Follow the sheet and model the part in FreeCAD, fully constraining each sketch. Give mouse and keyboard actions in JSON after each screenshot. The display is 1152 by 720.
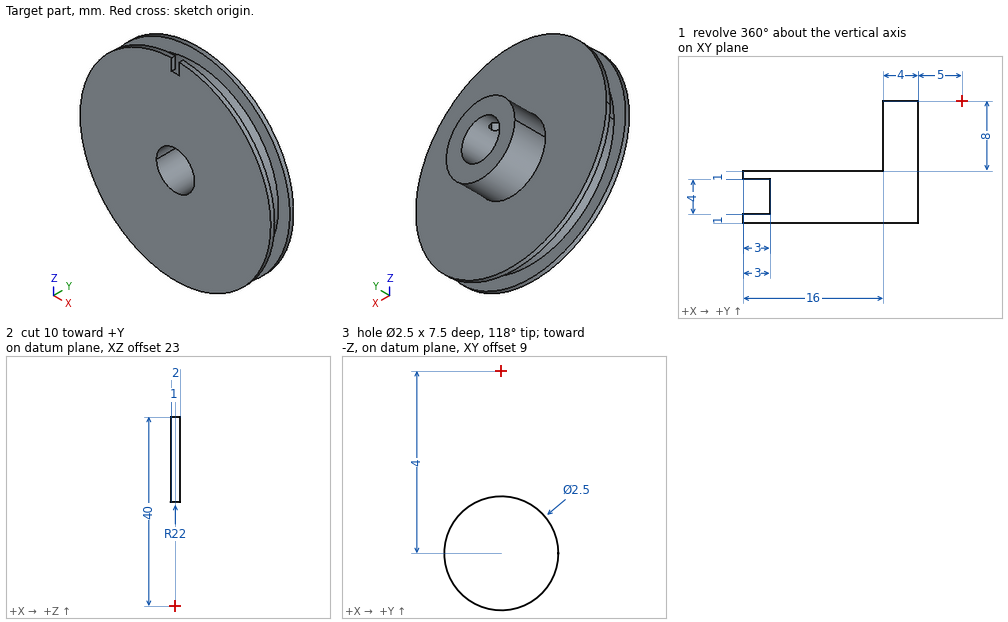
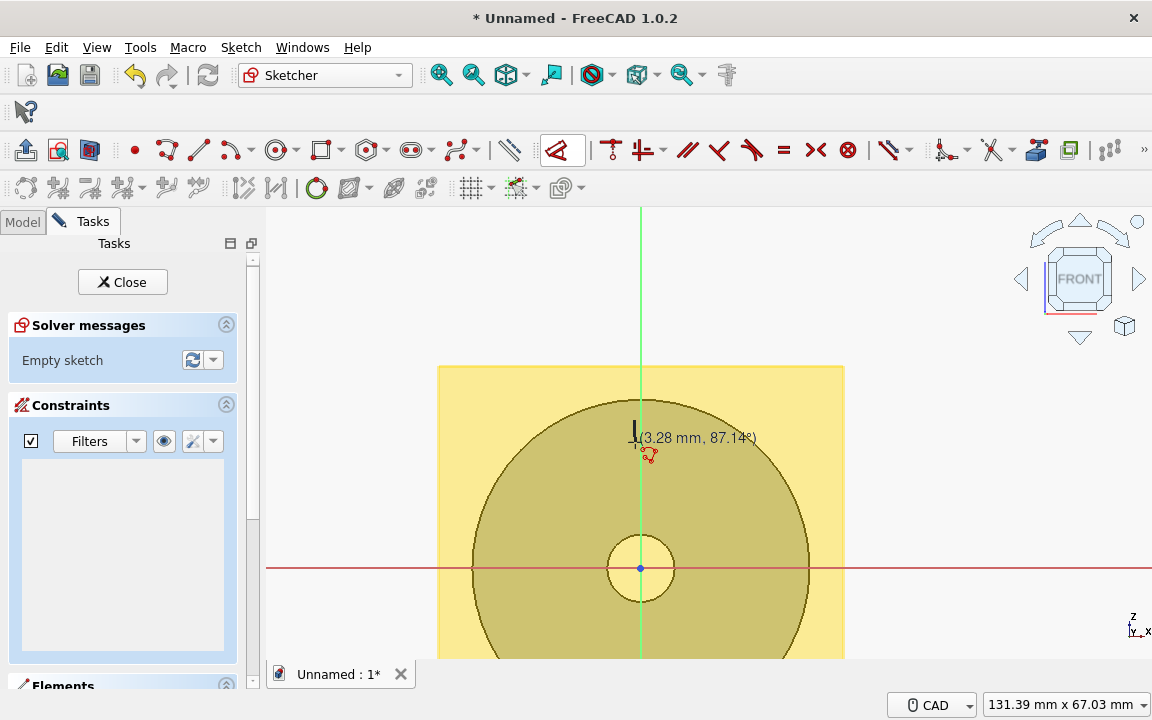
{"action": "scroll", "coordinate": [634, 299], "scroll_direction": "up", "scroll_amount": 5}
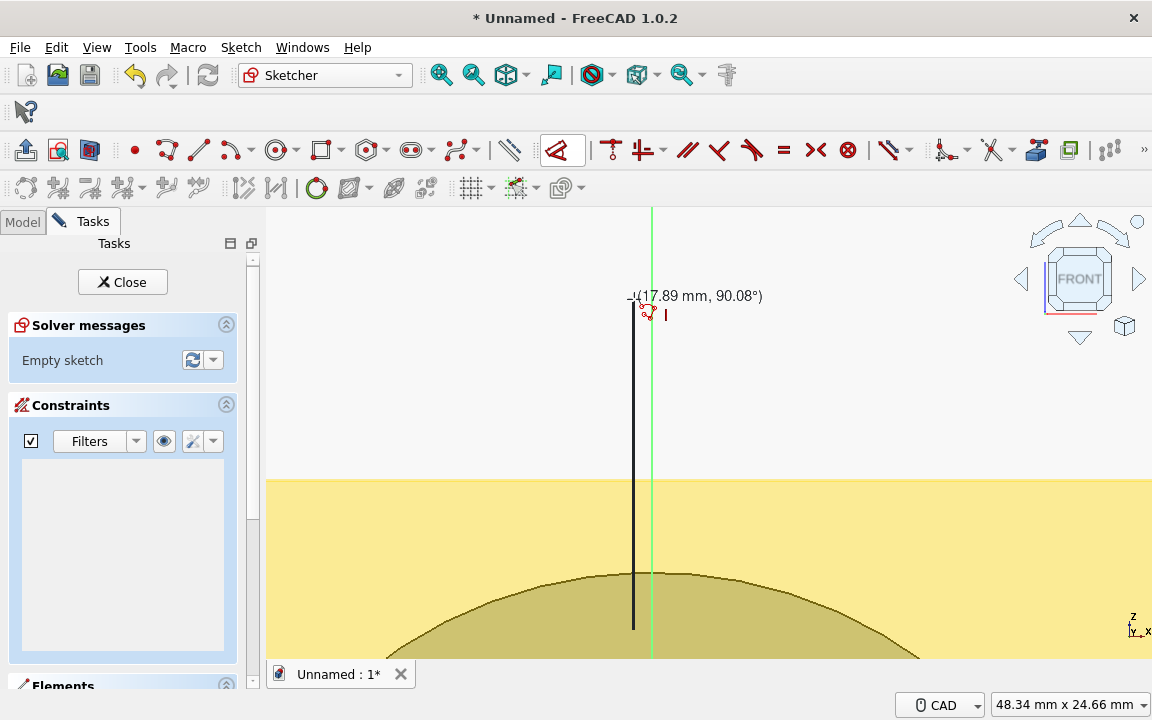
{"action": "left_click", "coordinate": [634, 298]}
{"action": "left_click", "coordinate": [670, 298]}
{"action": "left_click", "coordinate": [670, 628]}
{"action": "right_click", "coordinate": [670, 628]}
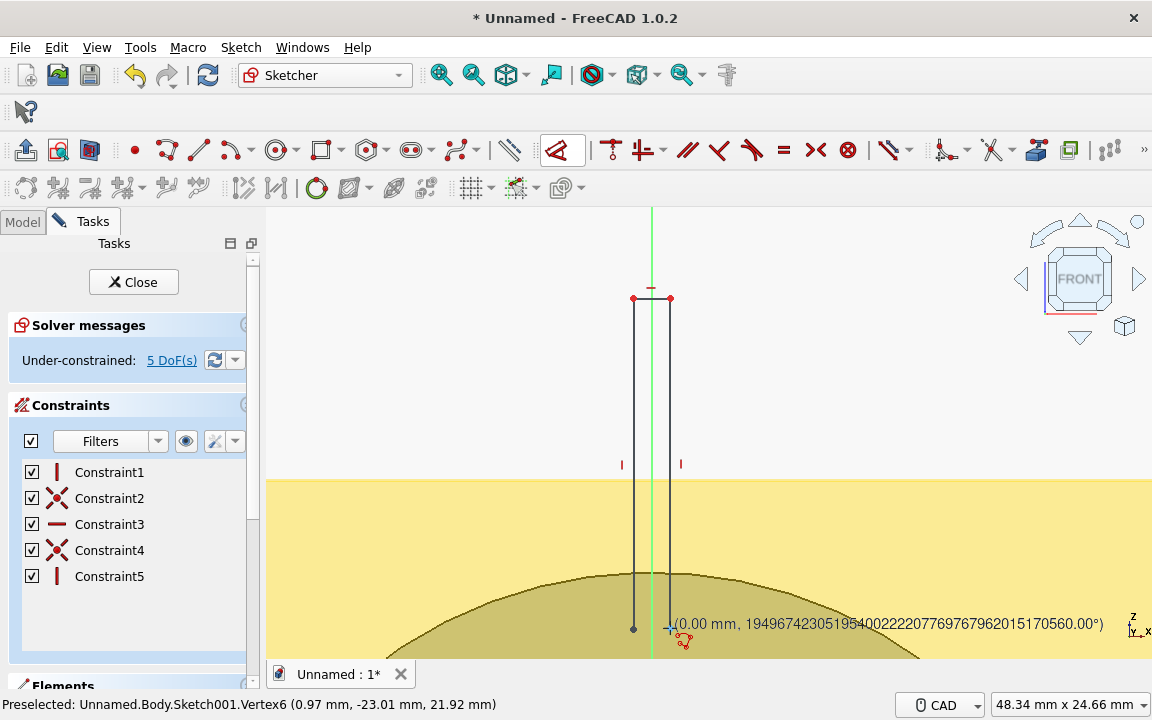
{"action": "key", "text": "g 3 a"}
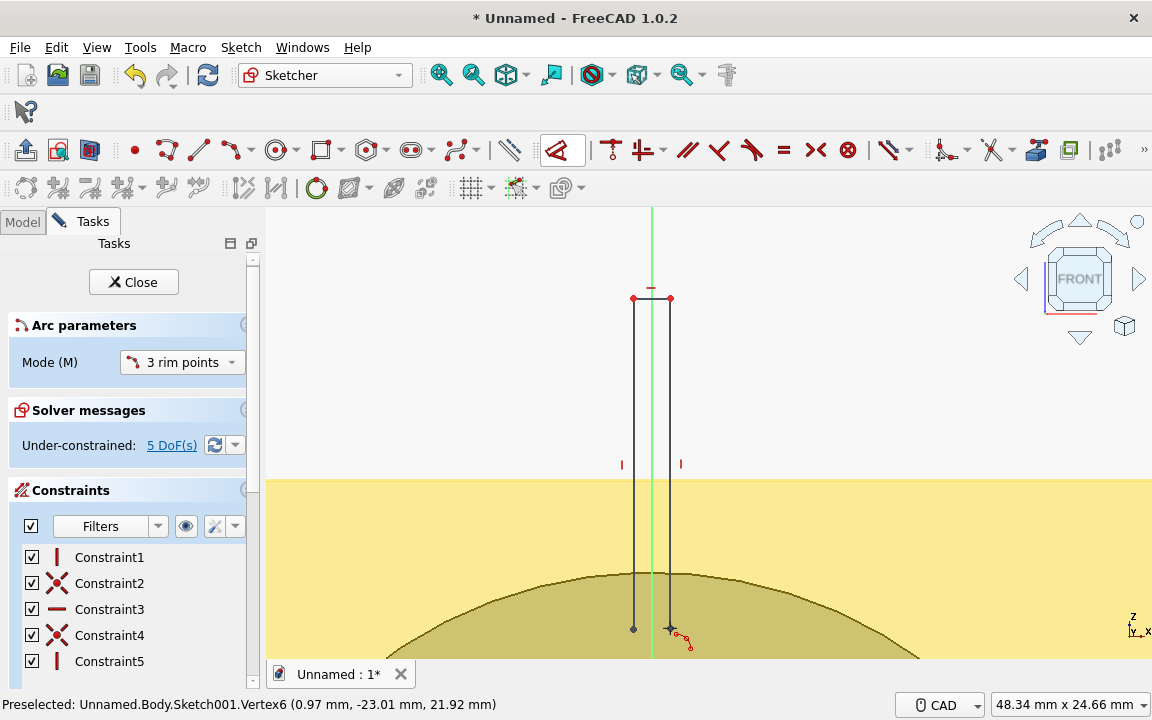
{"action": "left_click", "coordinate": [670, 629]}
{"action": "left_click", "coordinate": [634, 629]}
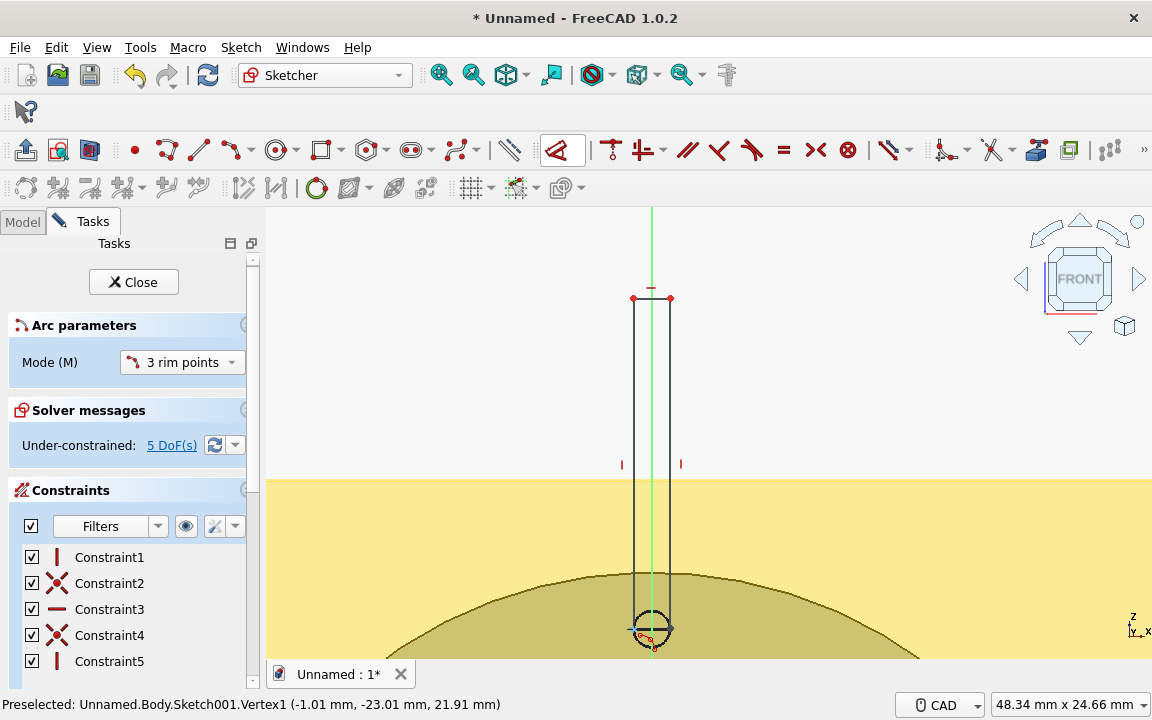
{"action": "scroll", "coordinate": [656, 628], "scroll_direction": "up", "scroll_amount": 19}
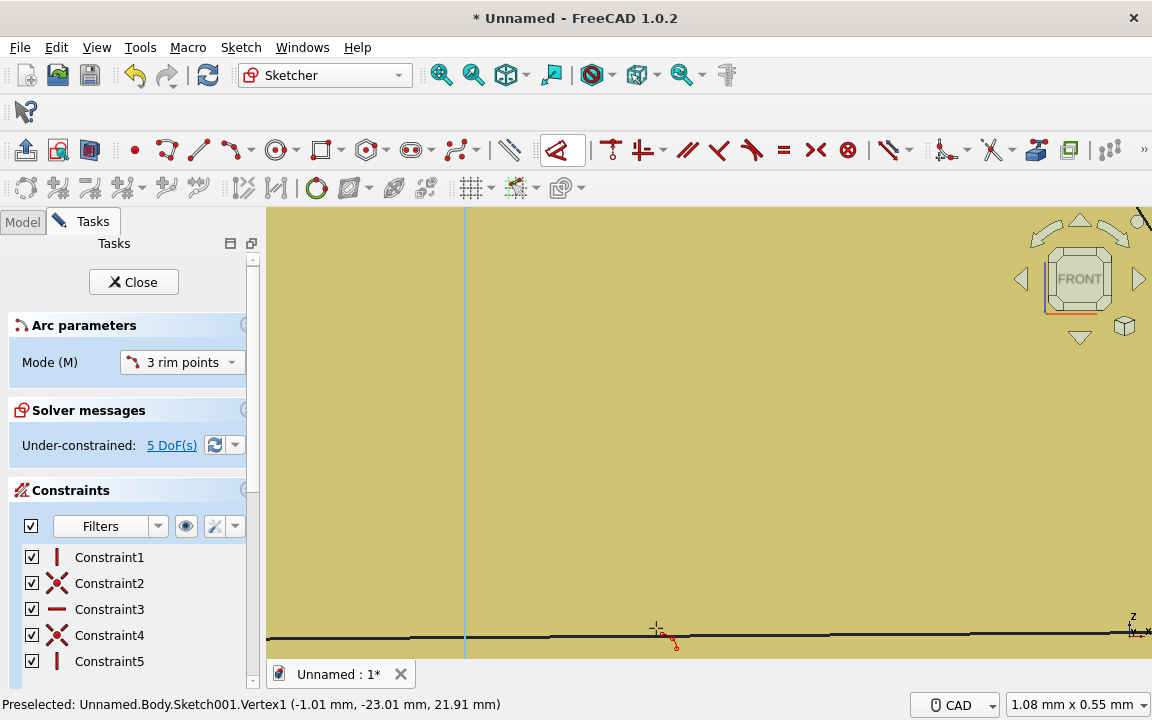
{"action": "left_click", "coordinate": [629, 570]}
{"action": "key", "text": "Escape"}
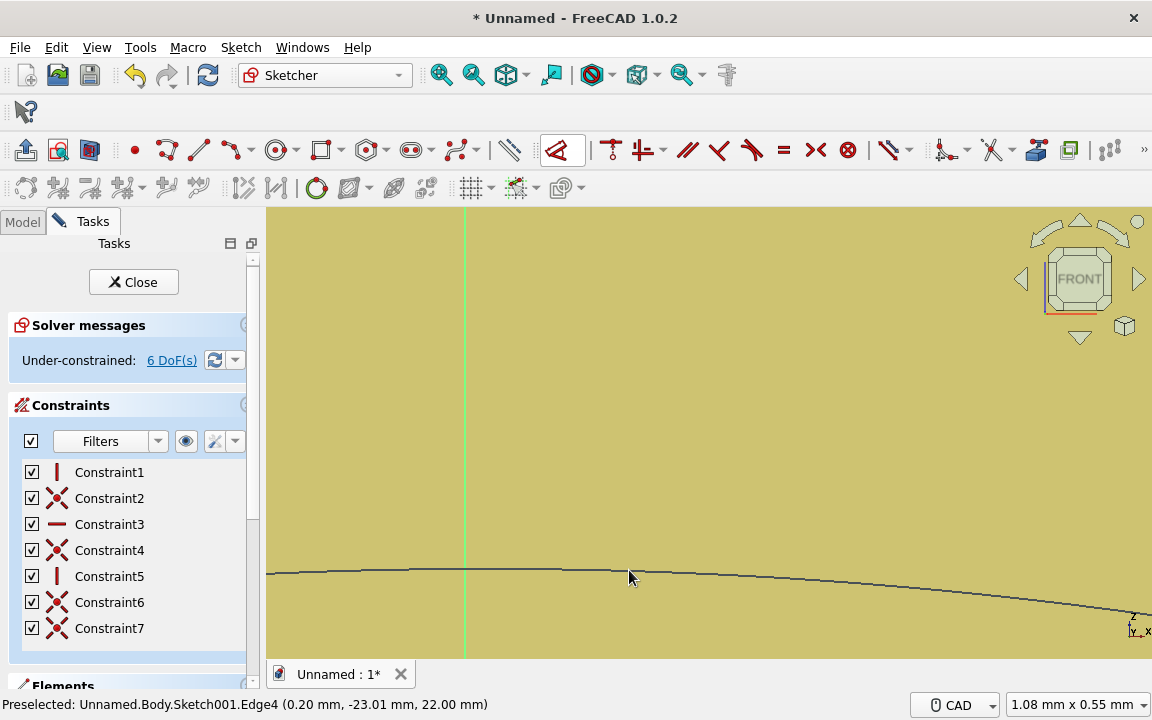
{"action": "scroll", "coordinate": [640, 433], "scroll_direction": "down", "scroll_amount": 15}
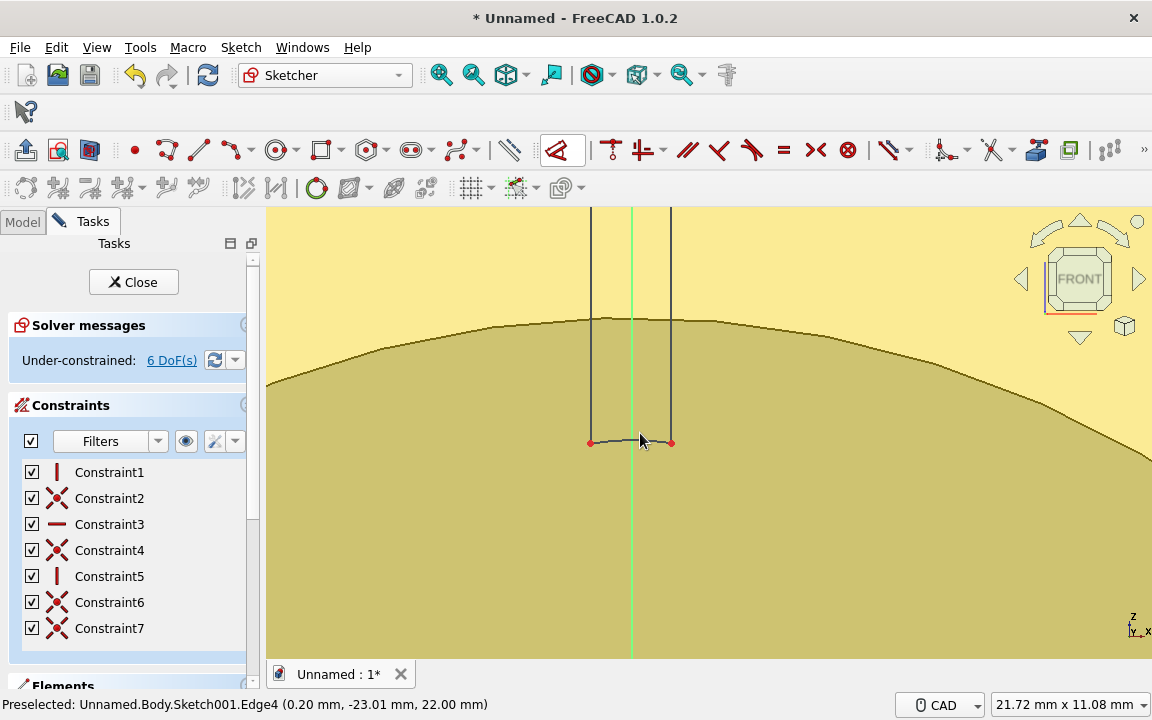
{"action": "scroll", "coordinate": [642, 415], "scroll_direction": "down", "scroll_amount": 9}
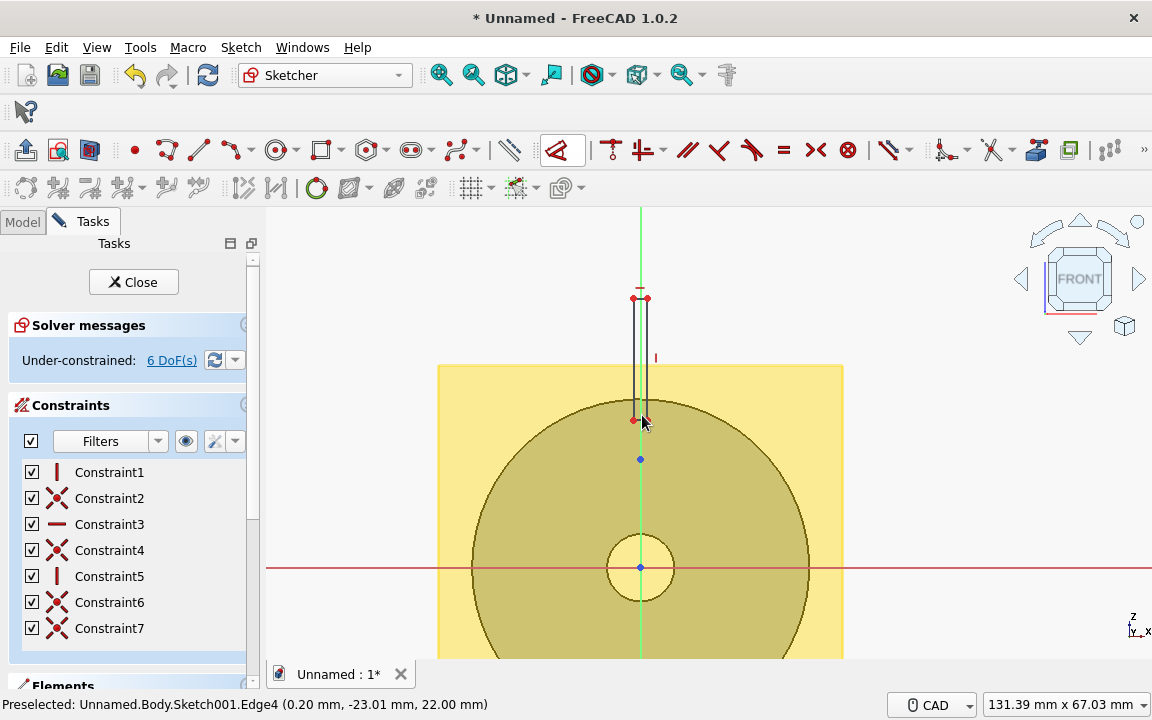
{"action": "left_click_drag", "start_coordinate": [631, 449], "coordinate": [651, 578]}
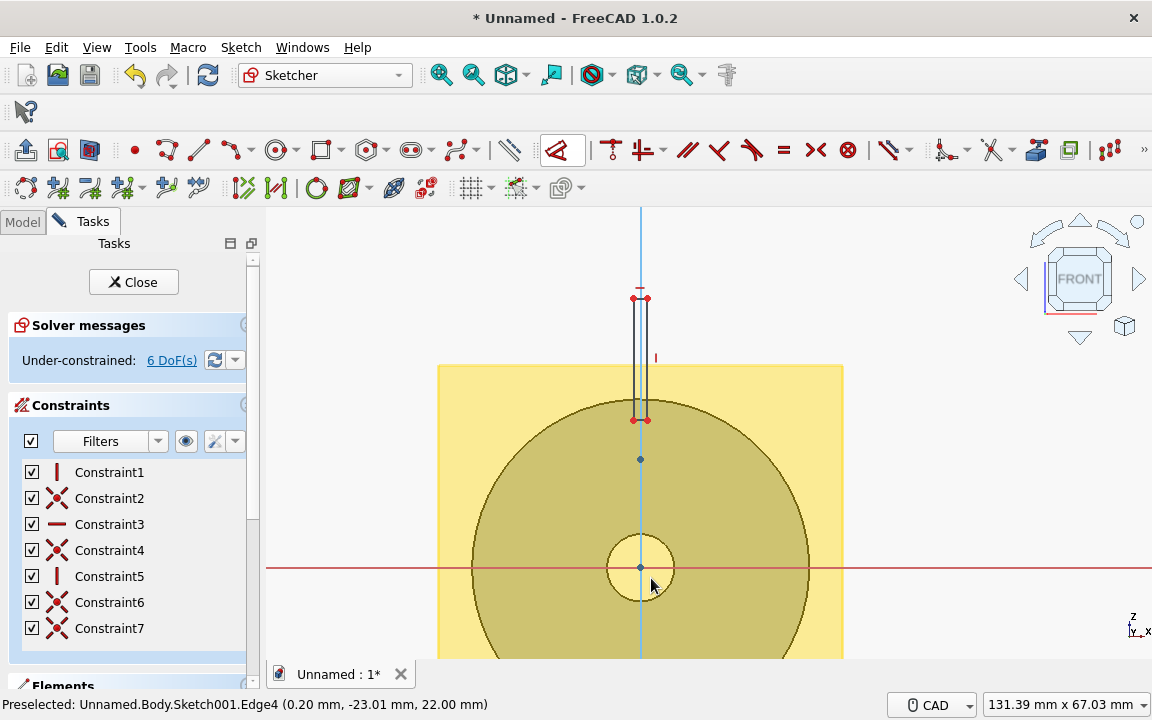
{"action": "key", "text": "c"}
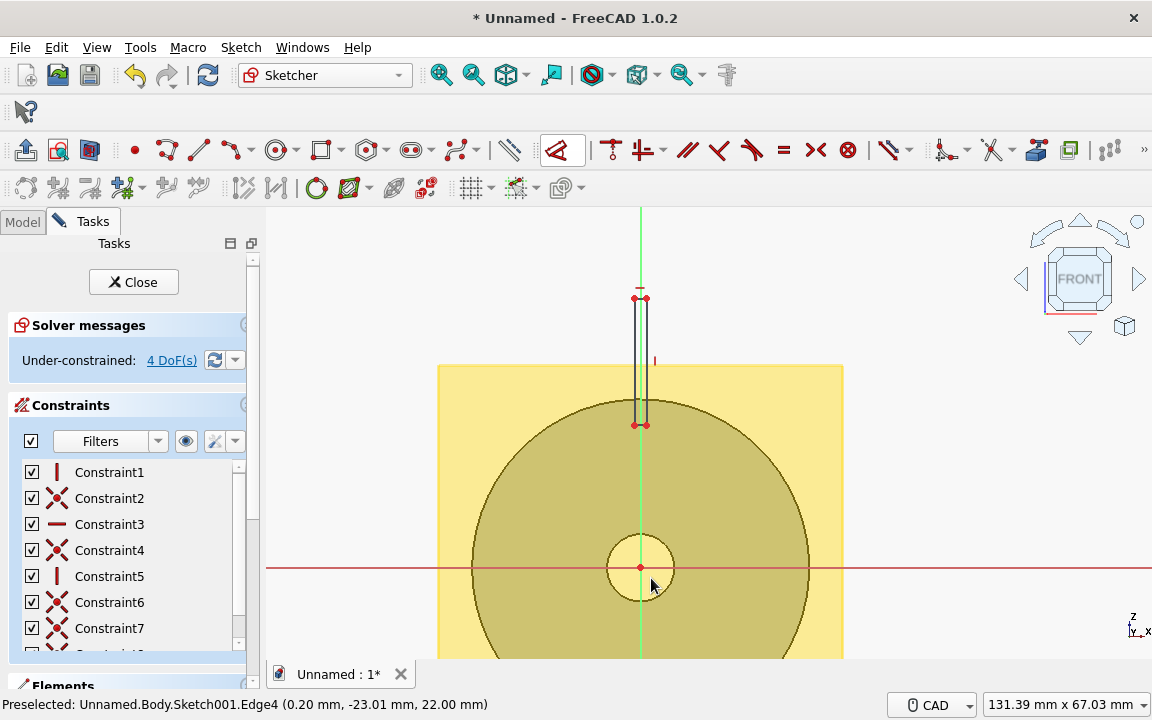
{"action": "scroll", "coordinate": [641, 425], "scroll_direction": "up", "scroll_amount": 5}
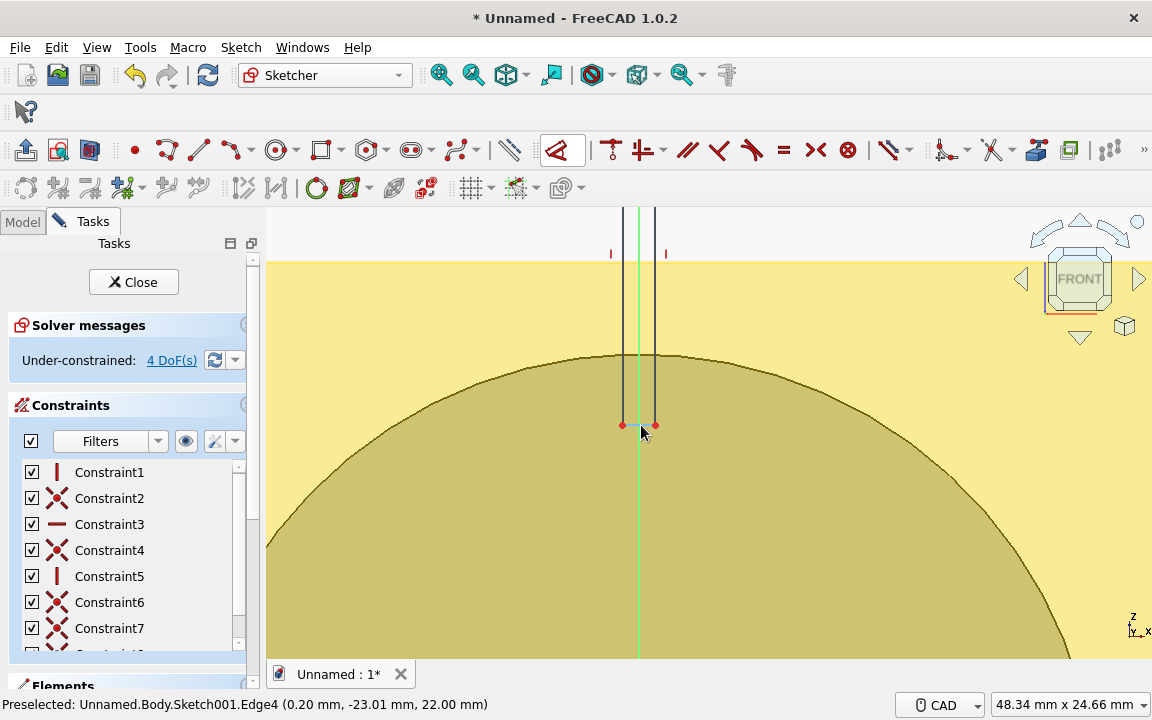
{"action": "left_click", "coordinate": [639, 425]}